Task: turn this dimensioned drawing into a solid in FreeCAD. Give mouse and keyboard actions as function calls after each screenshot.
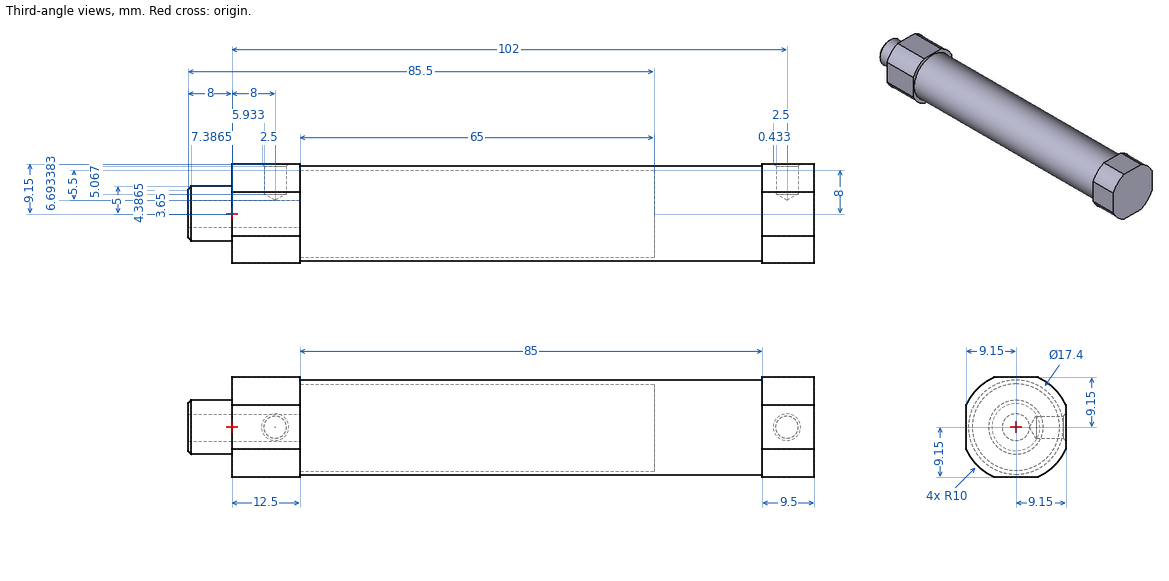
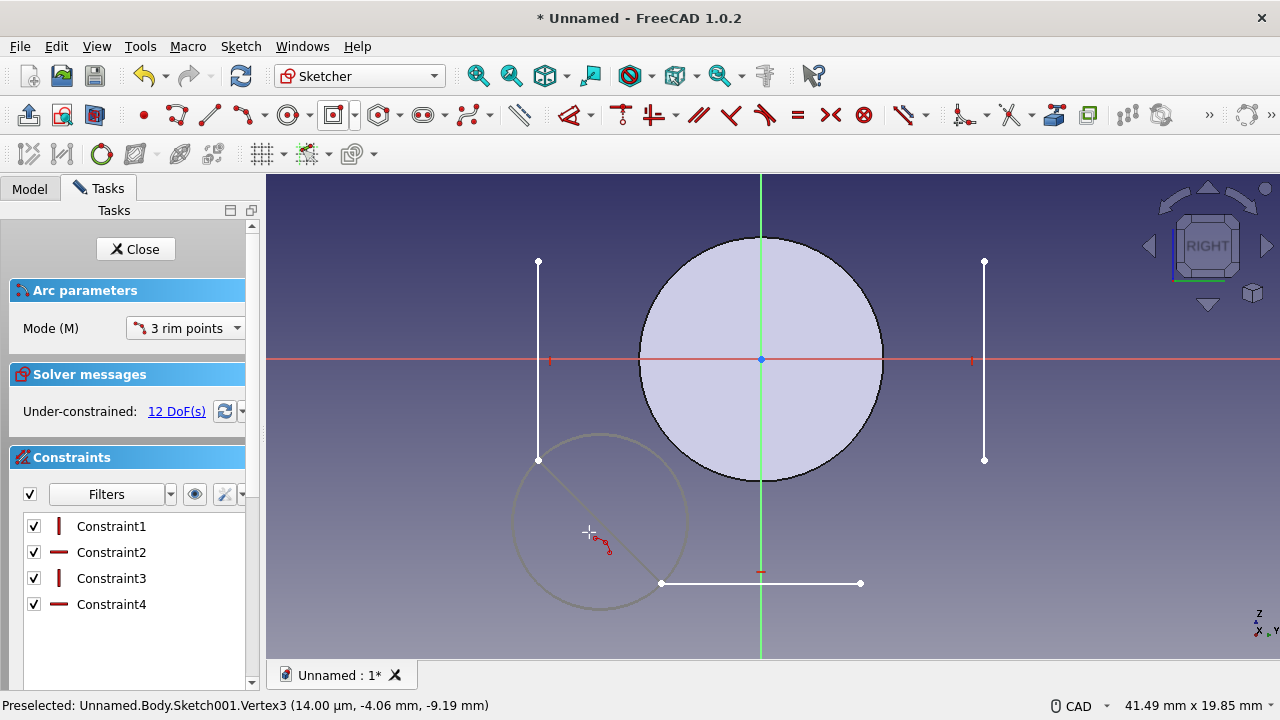
click(588, 532)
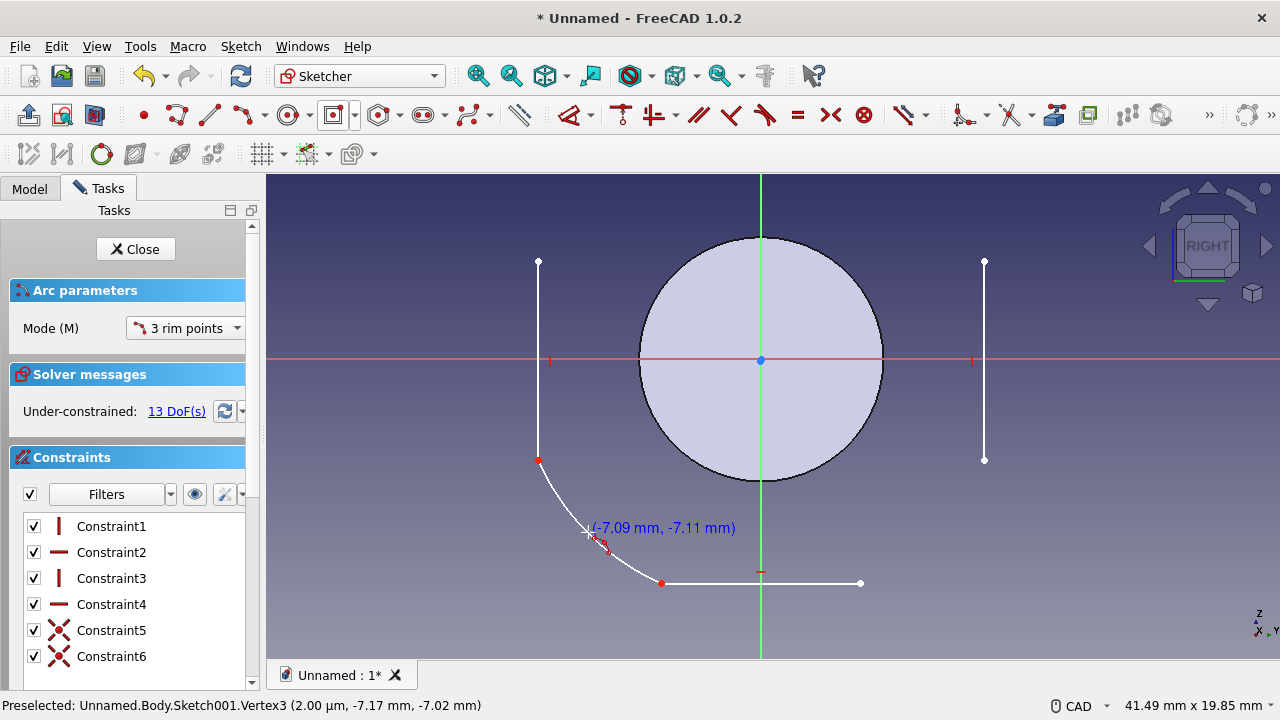
click(860, 584)
click(984, 460)
click(934, 532)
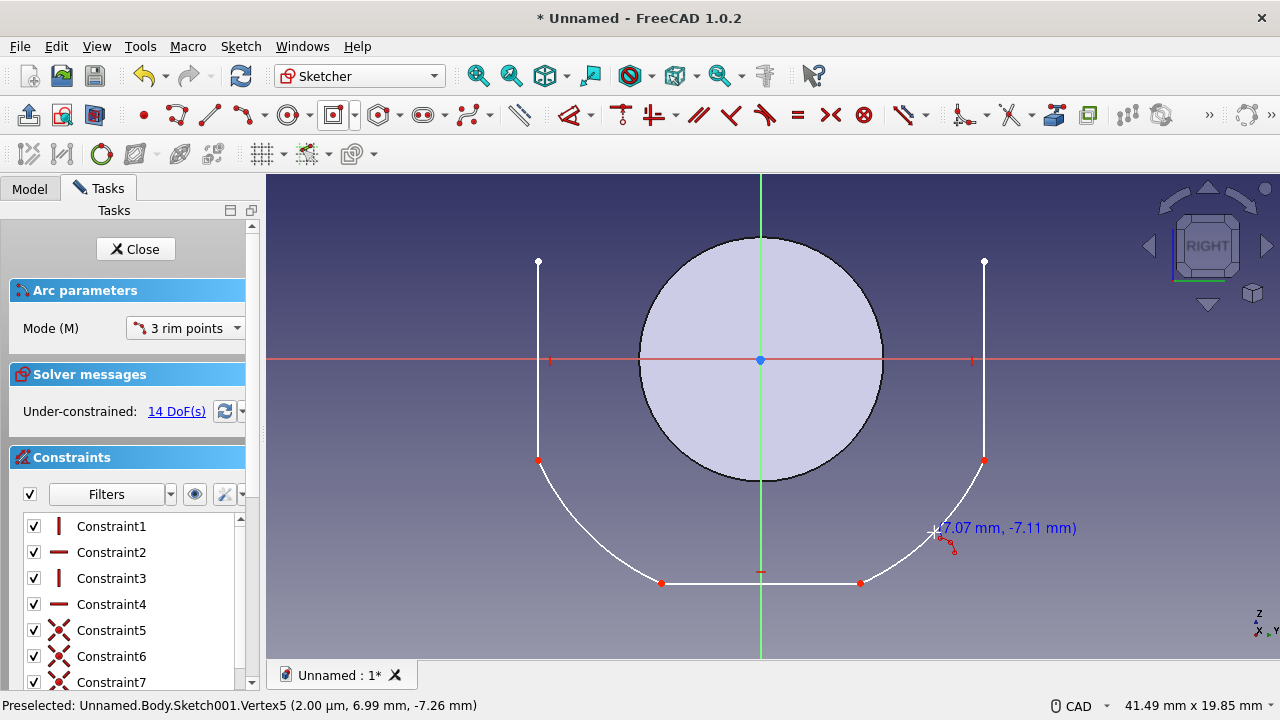
click(984, 262)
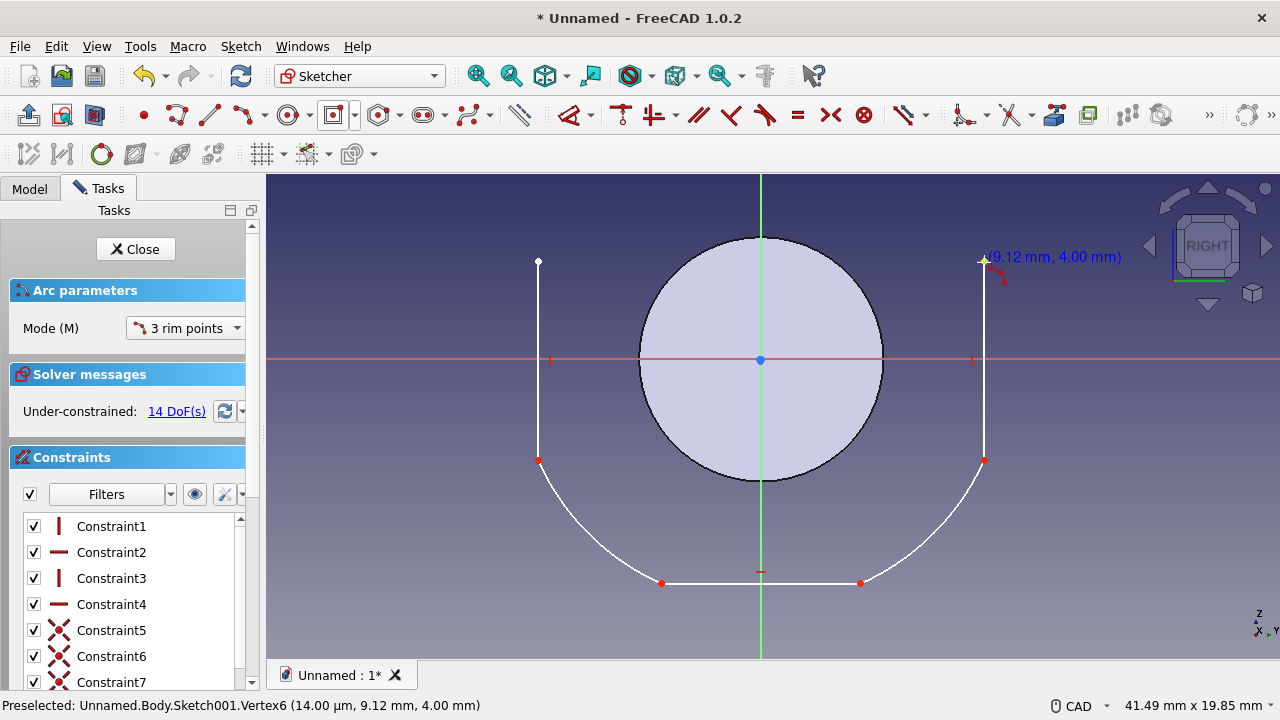
scroll(589, 533, down, 2)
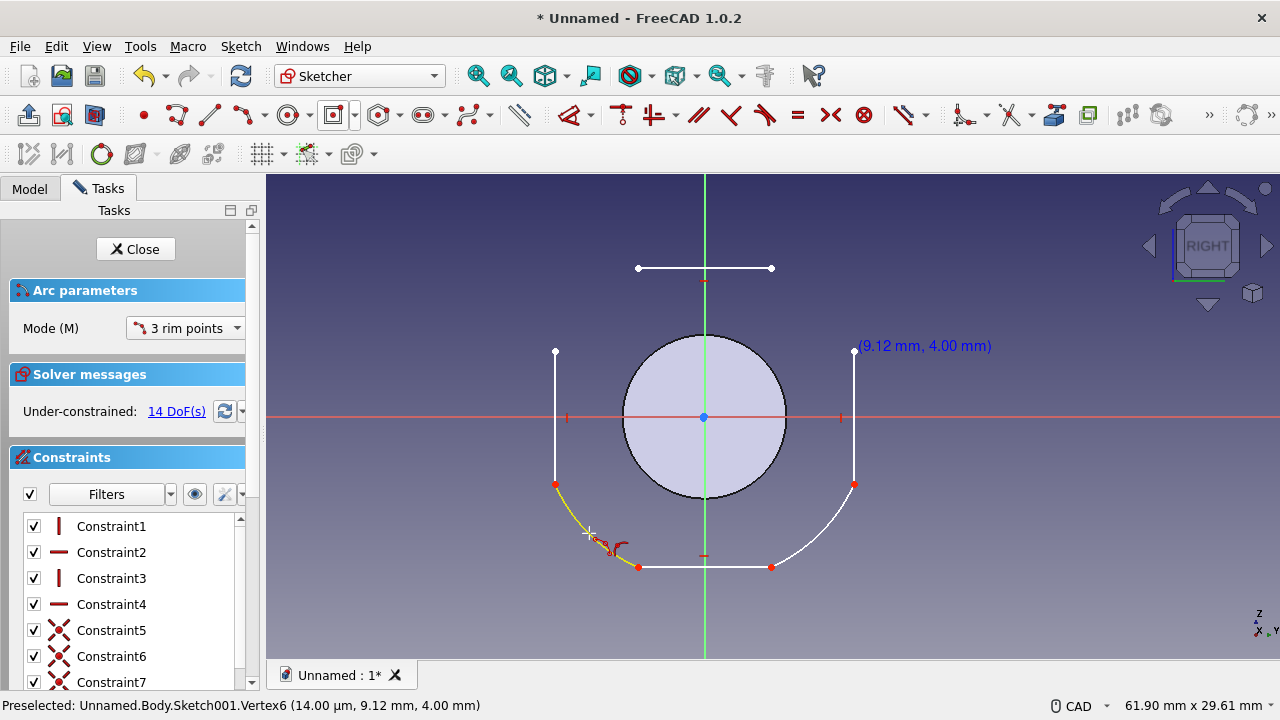
click(771, 268)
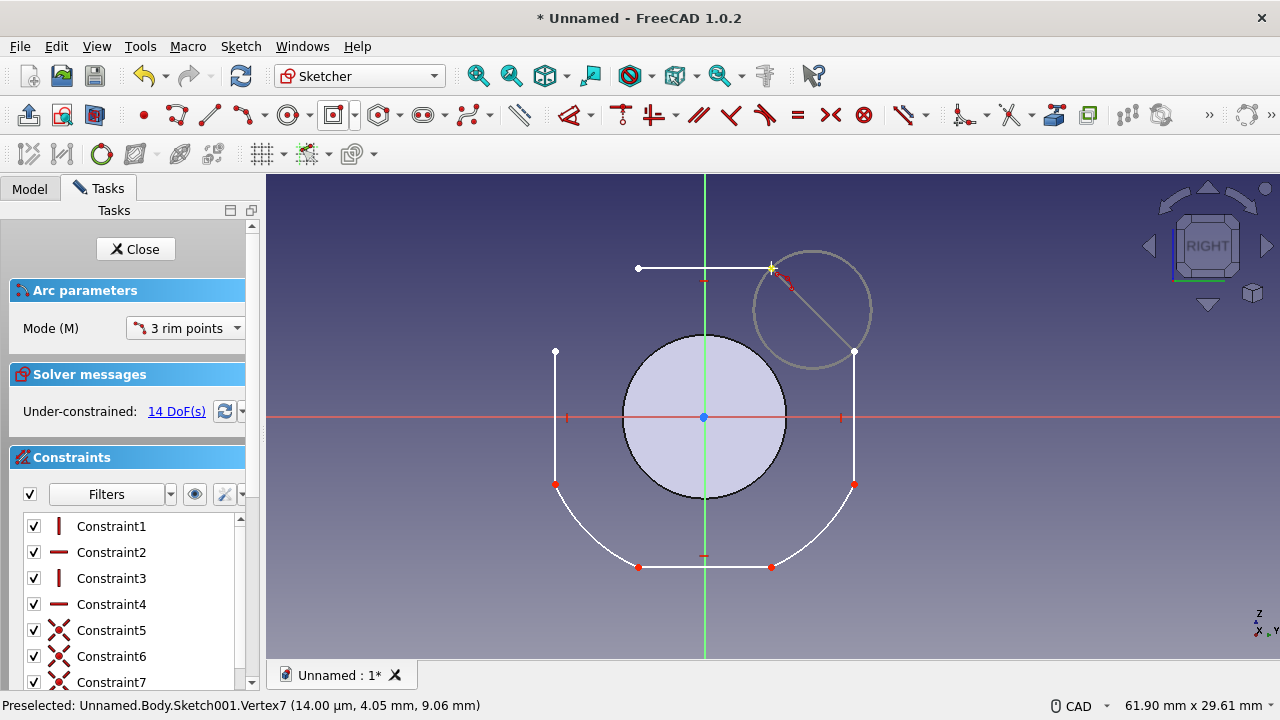
scroll(820, 301, up, 2)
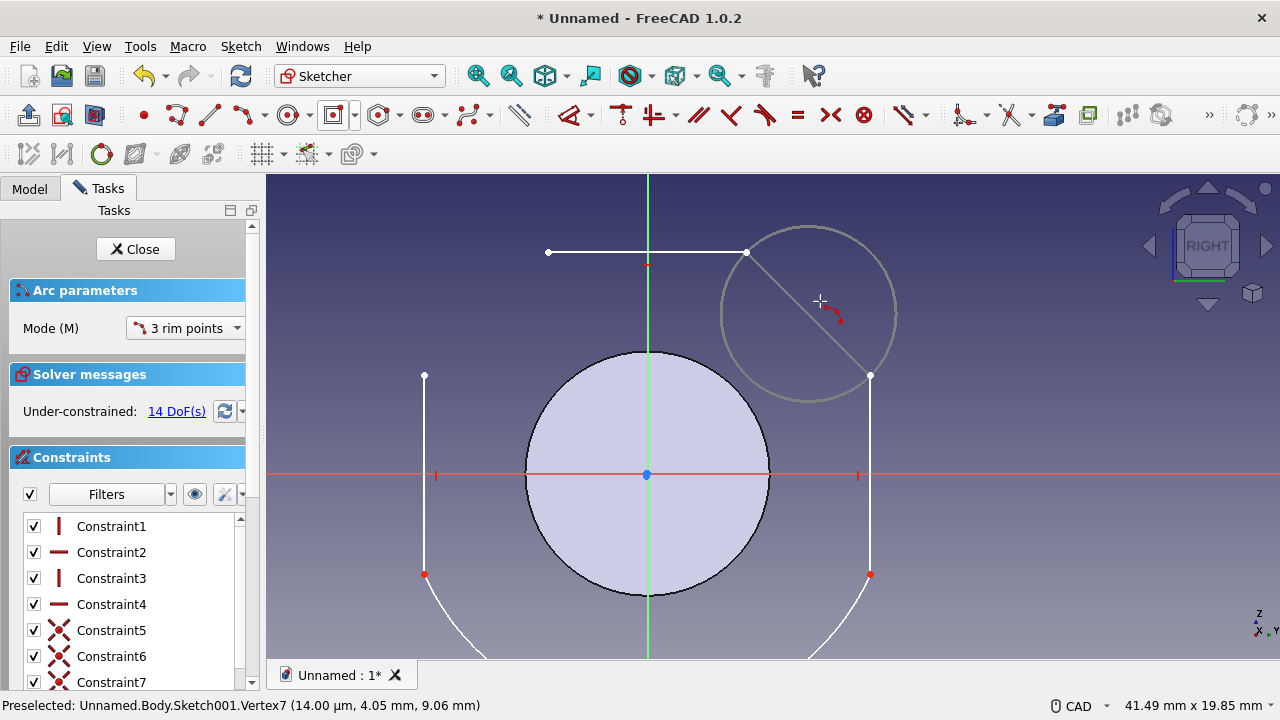
click(820, 301)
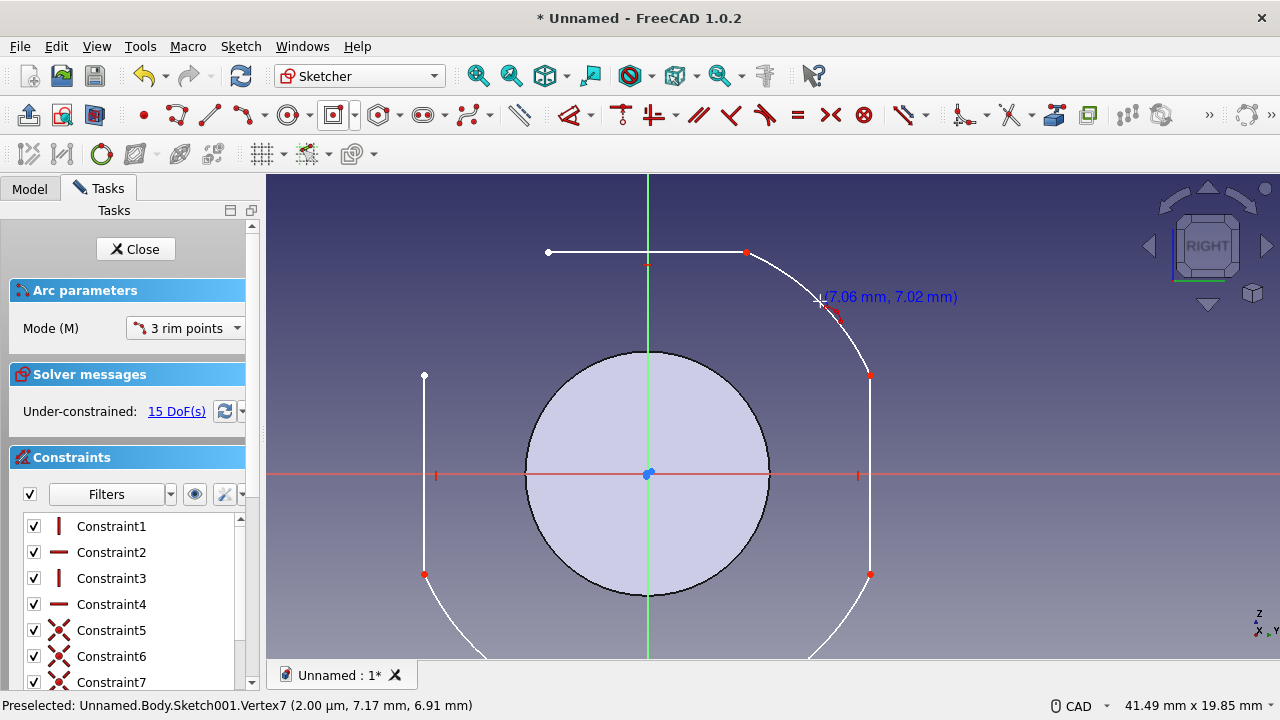
click(548, 252)
click(424, 376)
click(475, 301)
key(Escape)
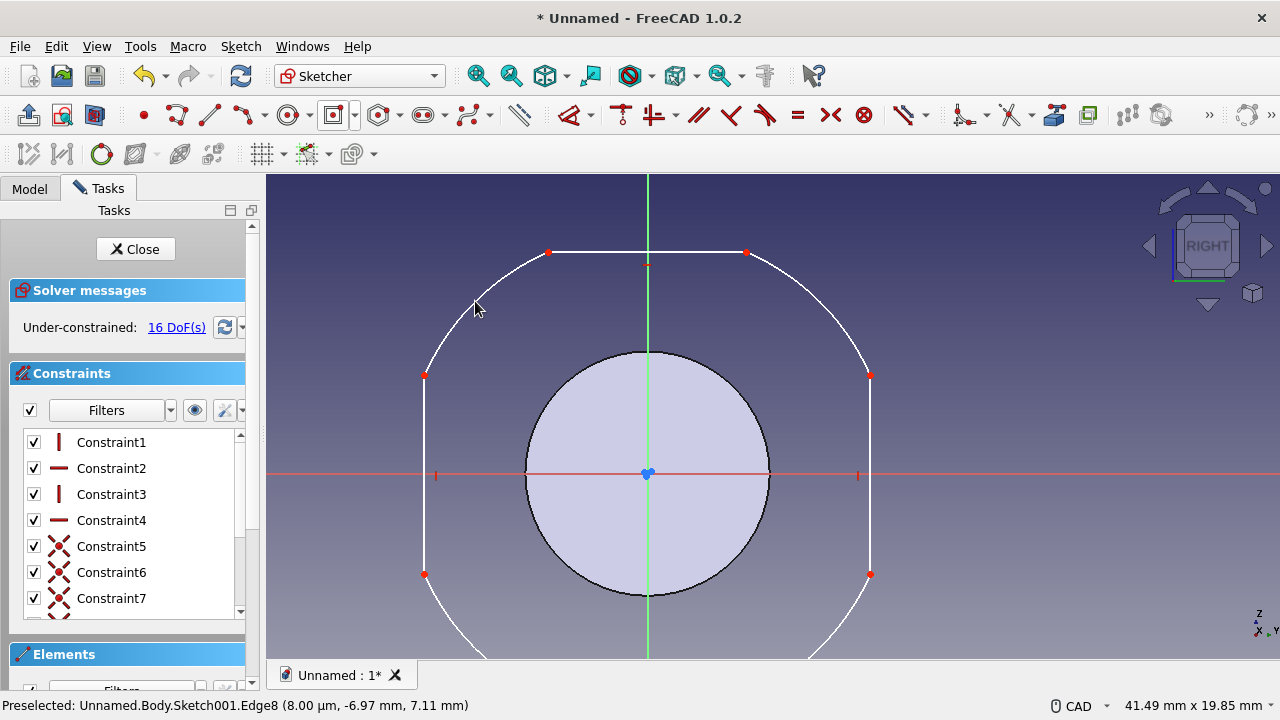
click(451, 621)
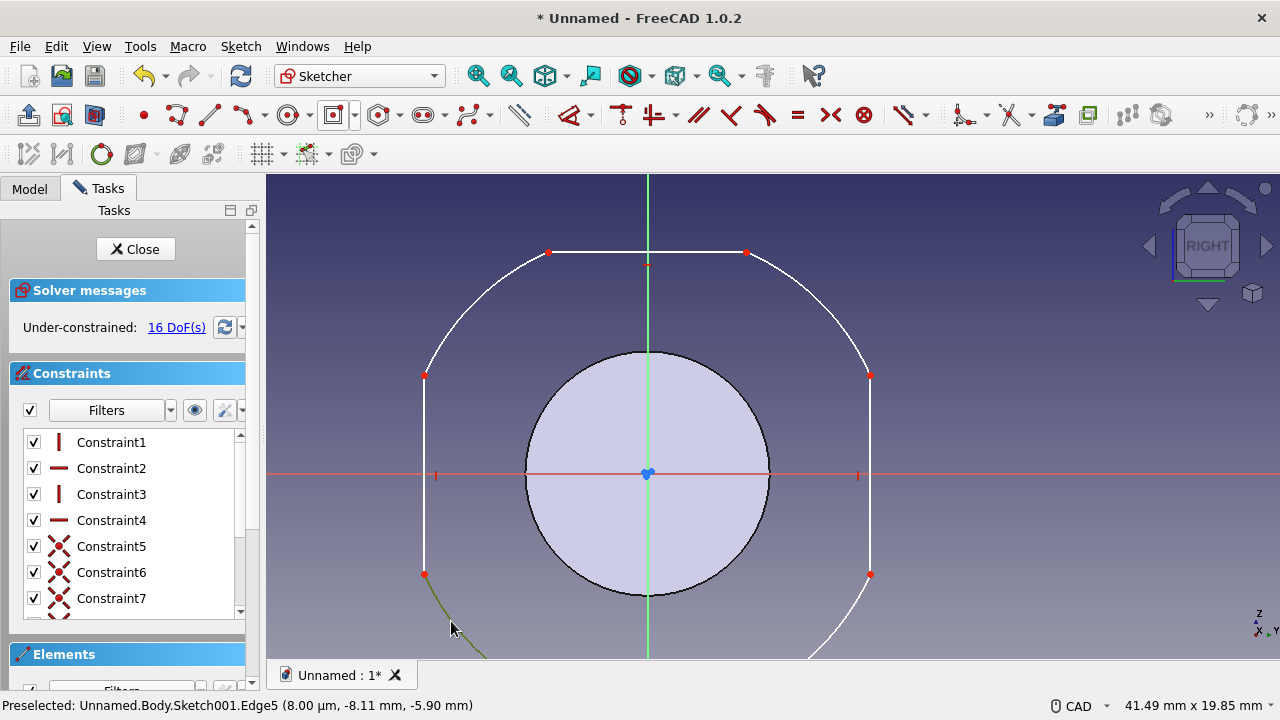
click(843, 621)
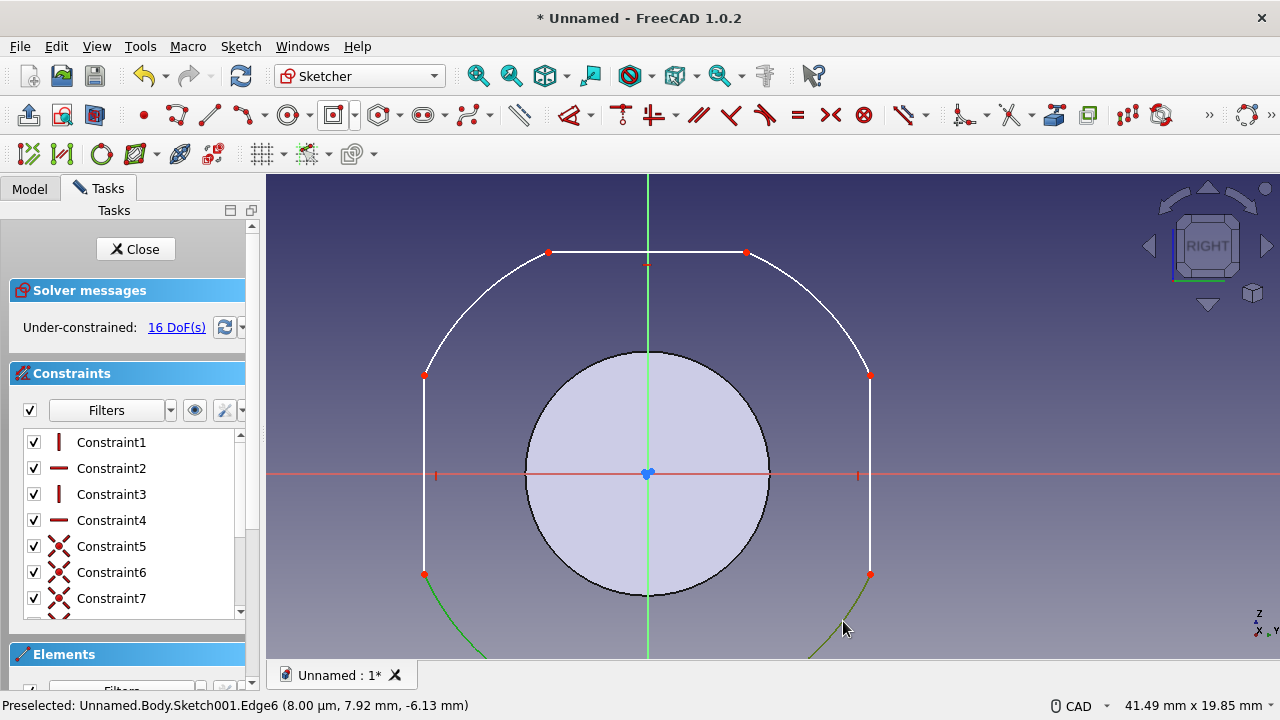
click(621, 116)